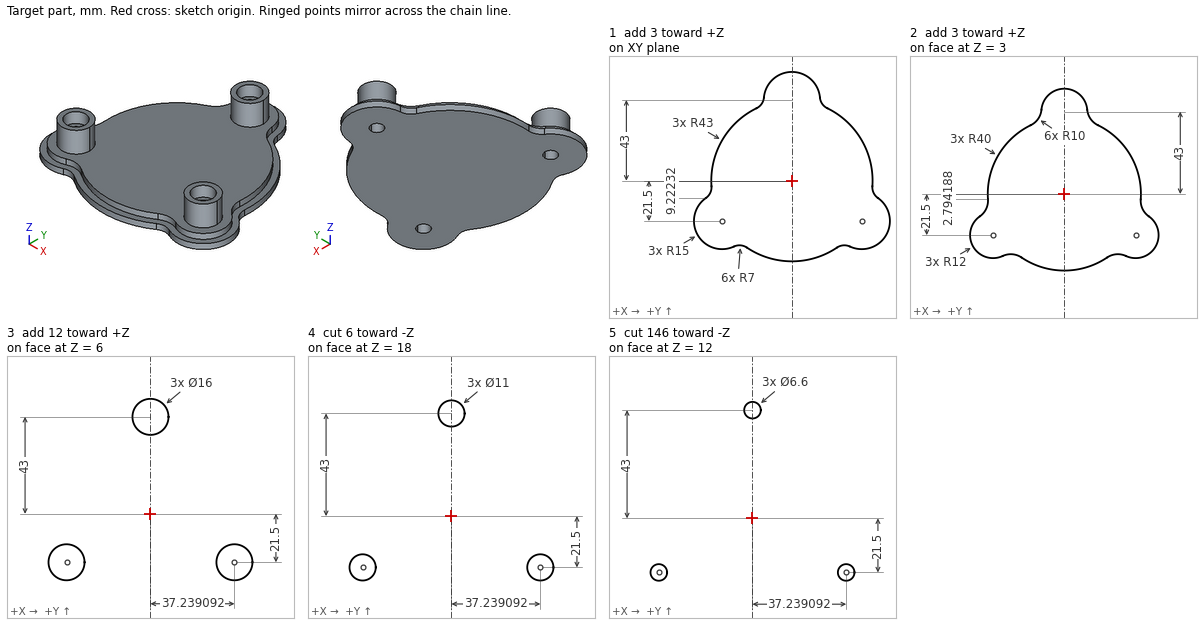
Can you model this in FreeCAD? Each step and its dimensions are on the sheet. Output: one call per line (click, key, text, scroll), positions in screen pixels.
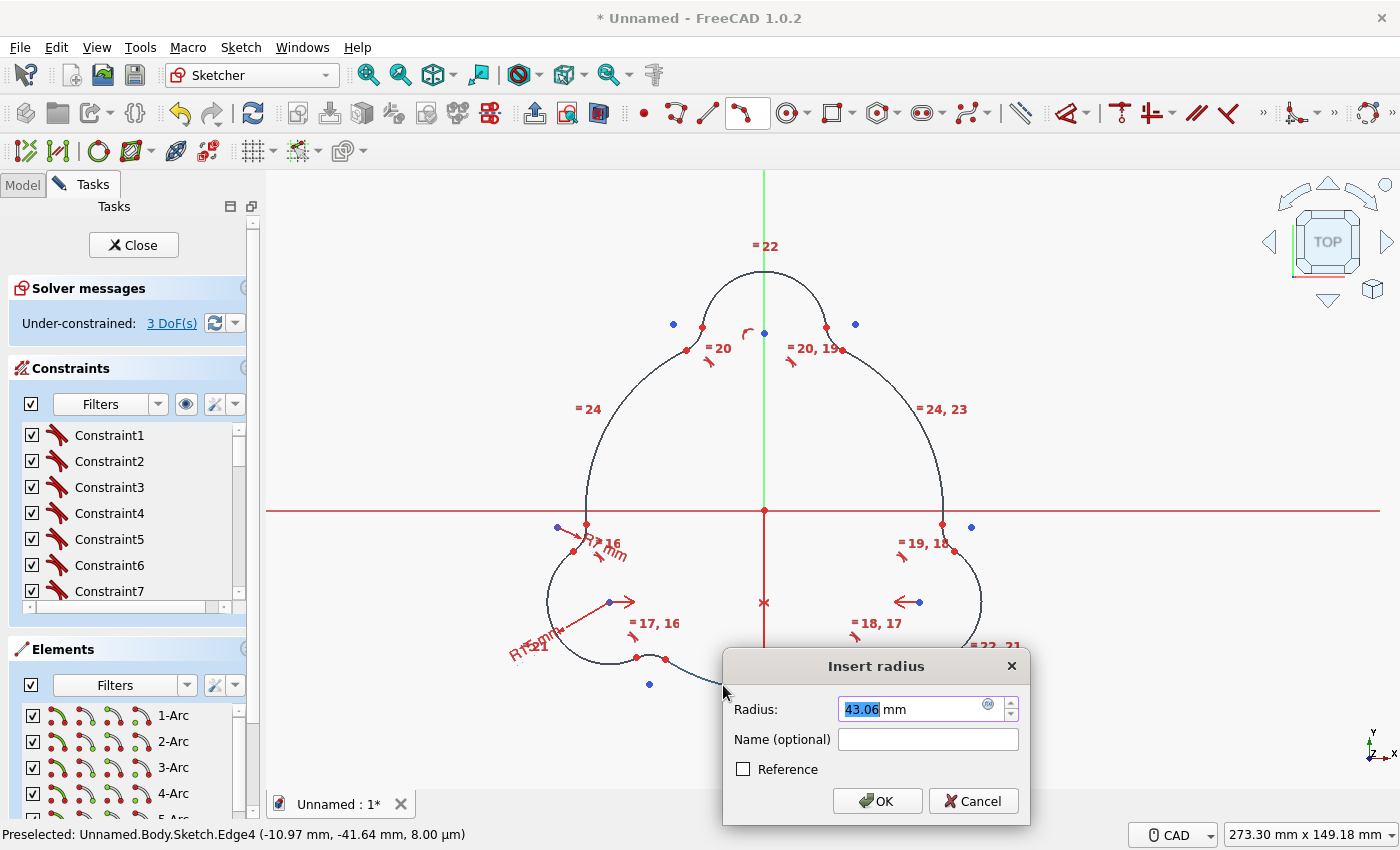
text(43)
key(Return)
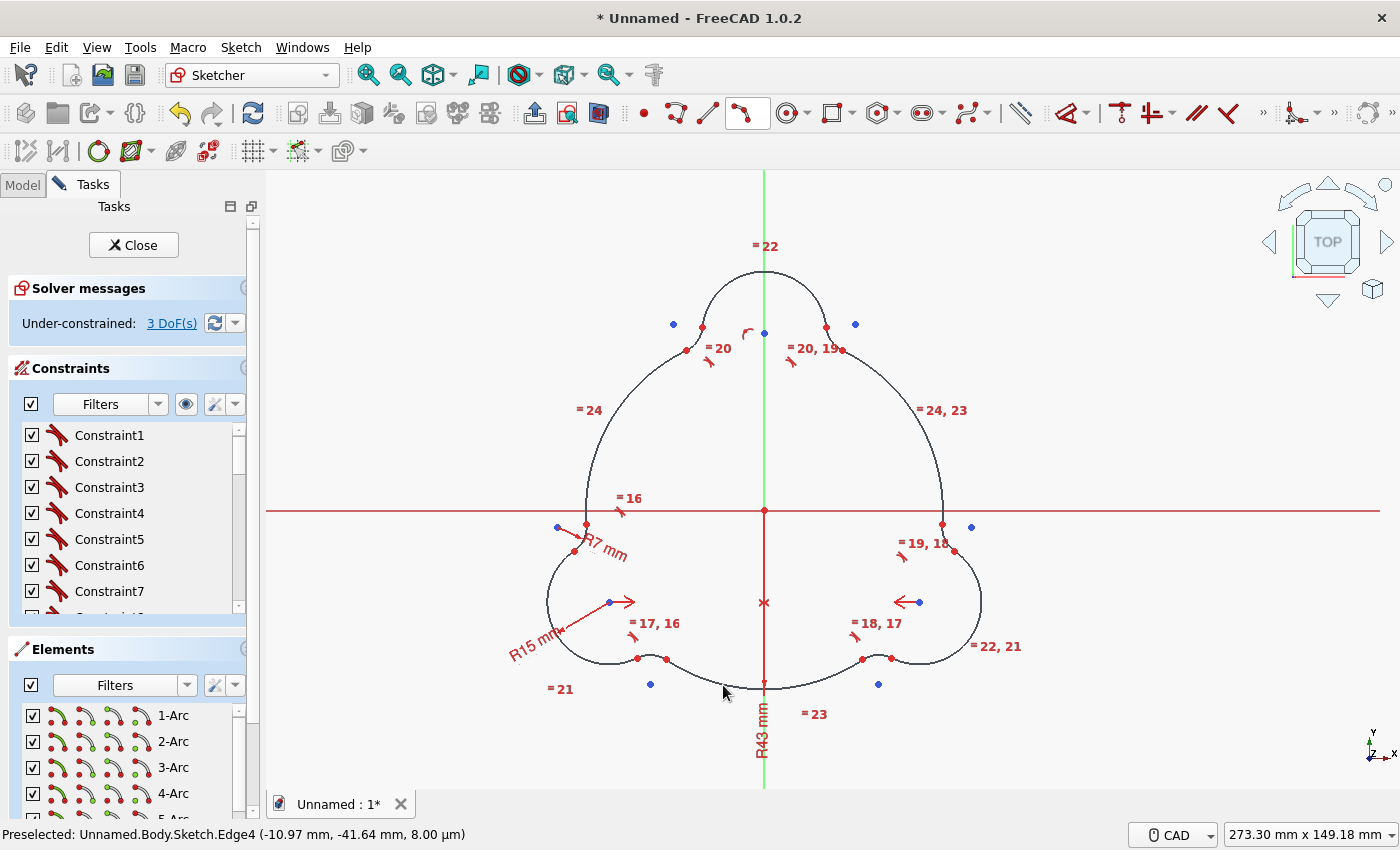
click(764, 334)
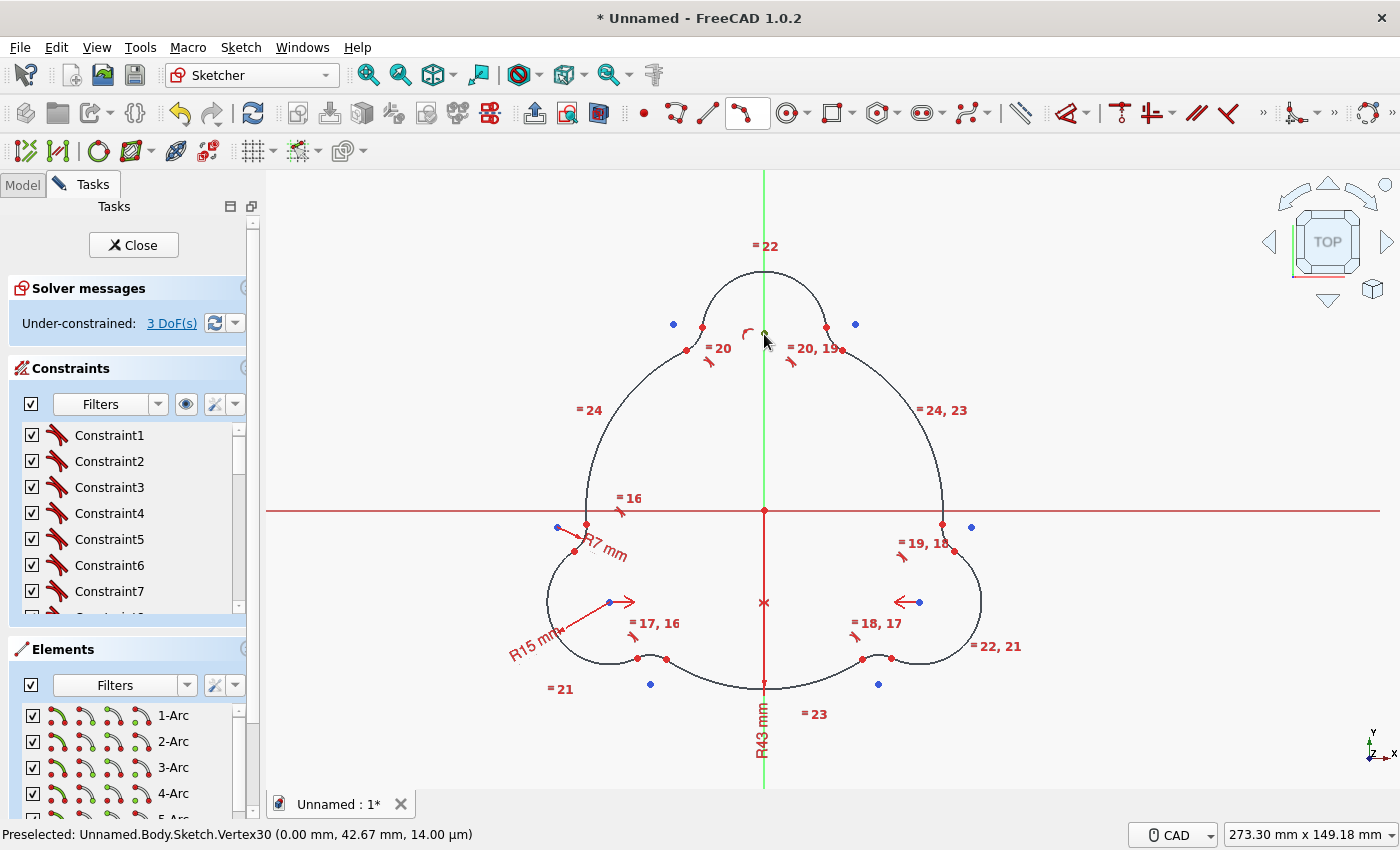
key(i)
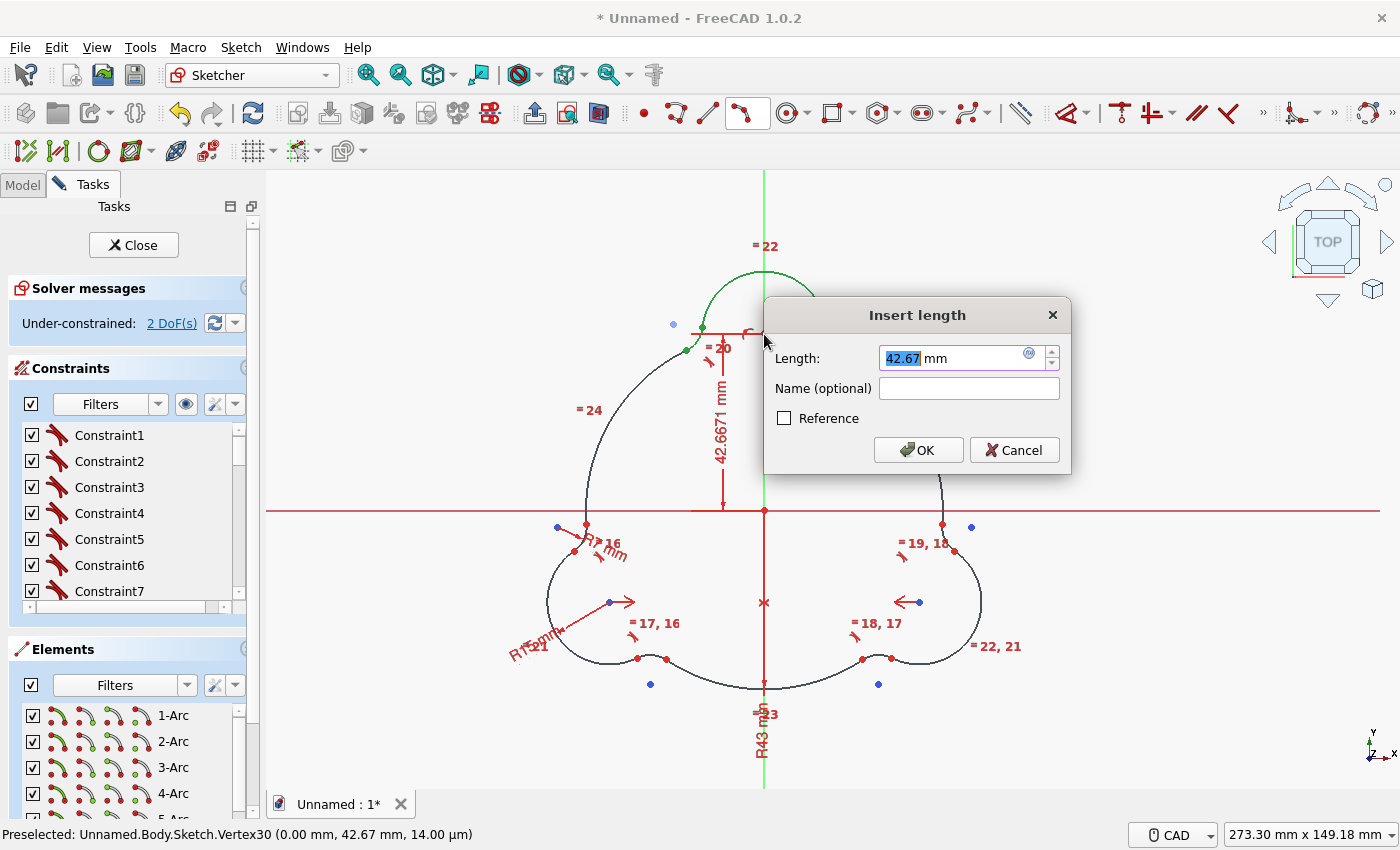
text(43)
key(Return)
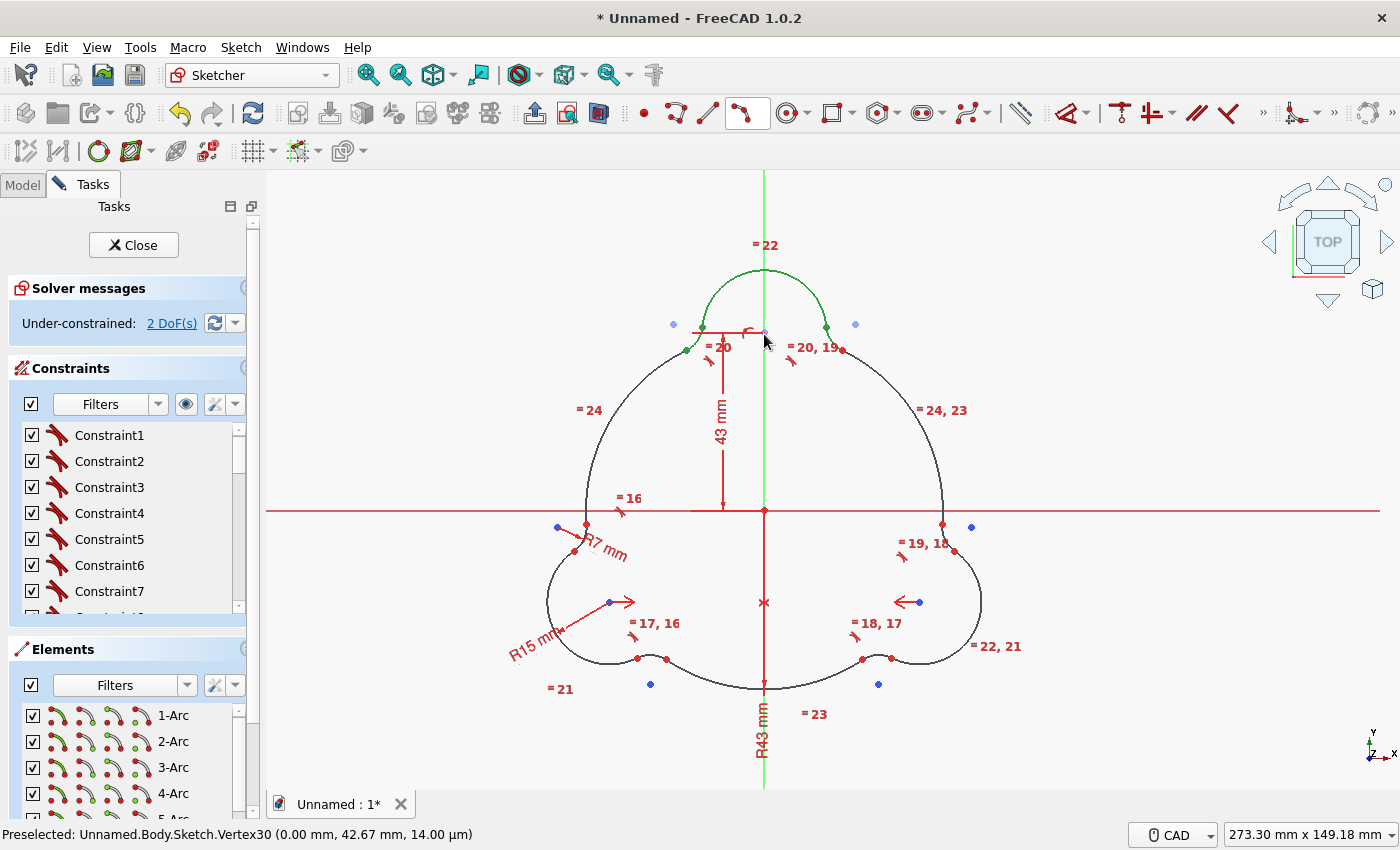
click(610, 602)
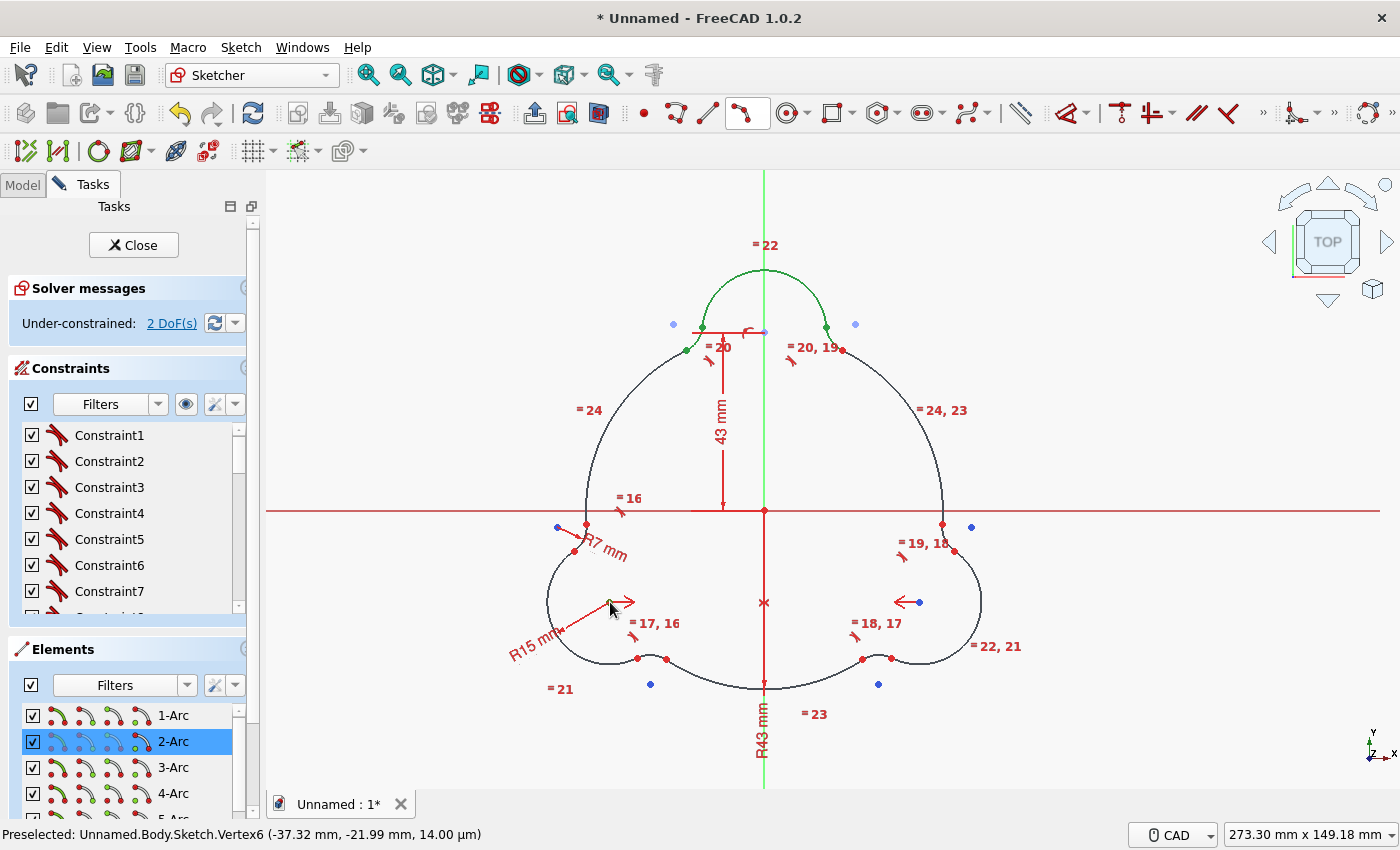
click(1088, 114)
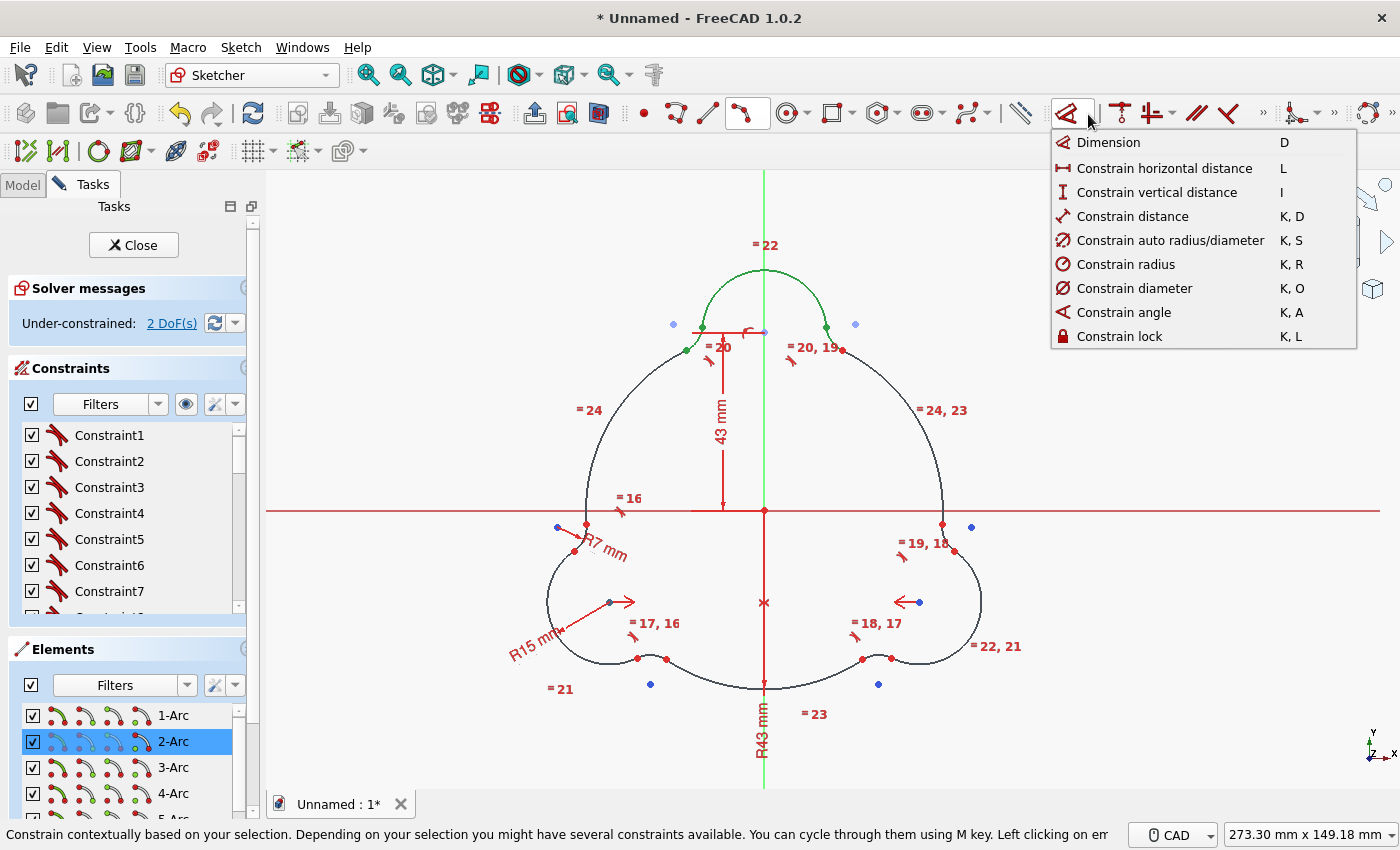
click(1204, 192)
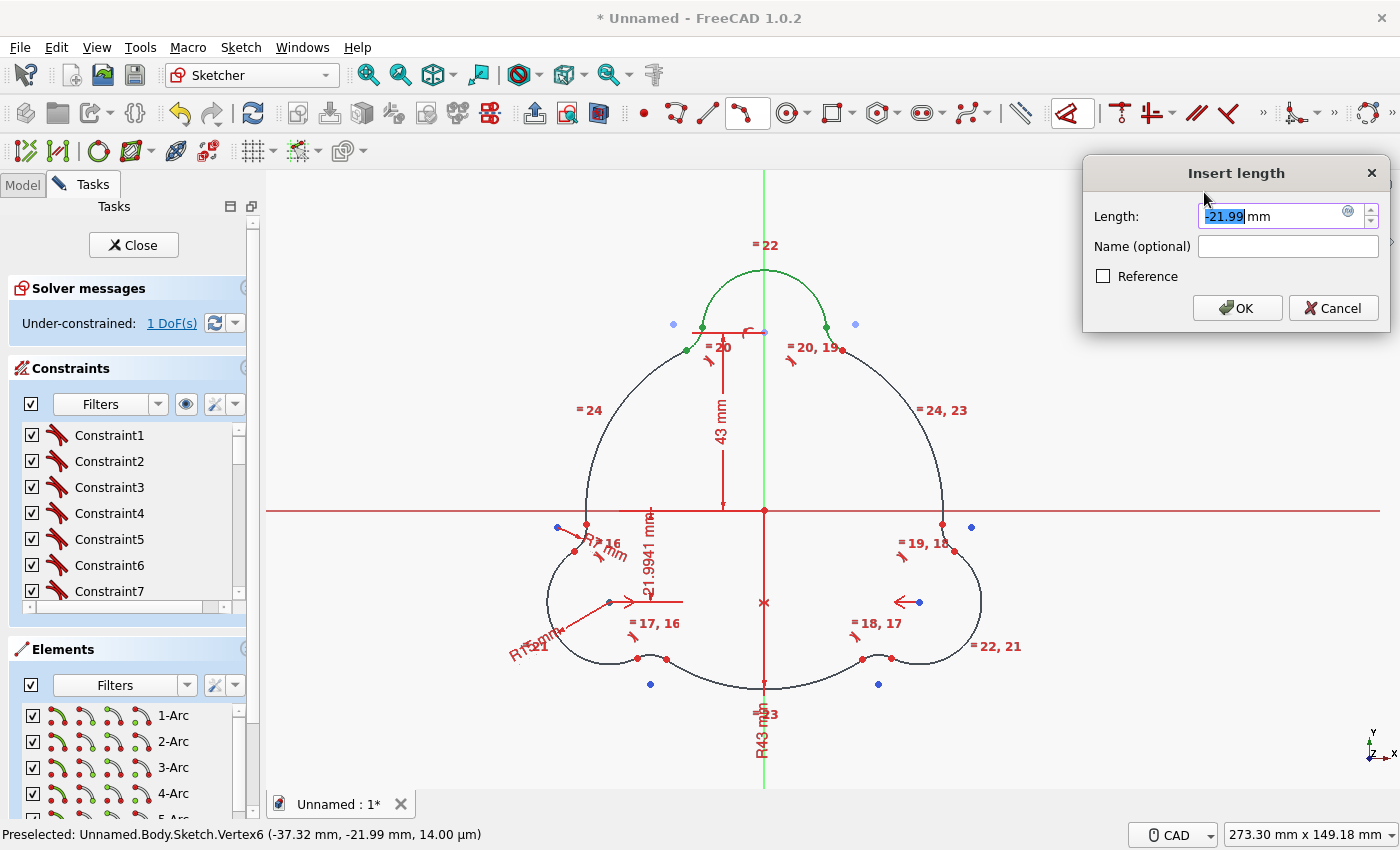
text(-21.5)
key(Return)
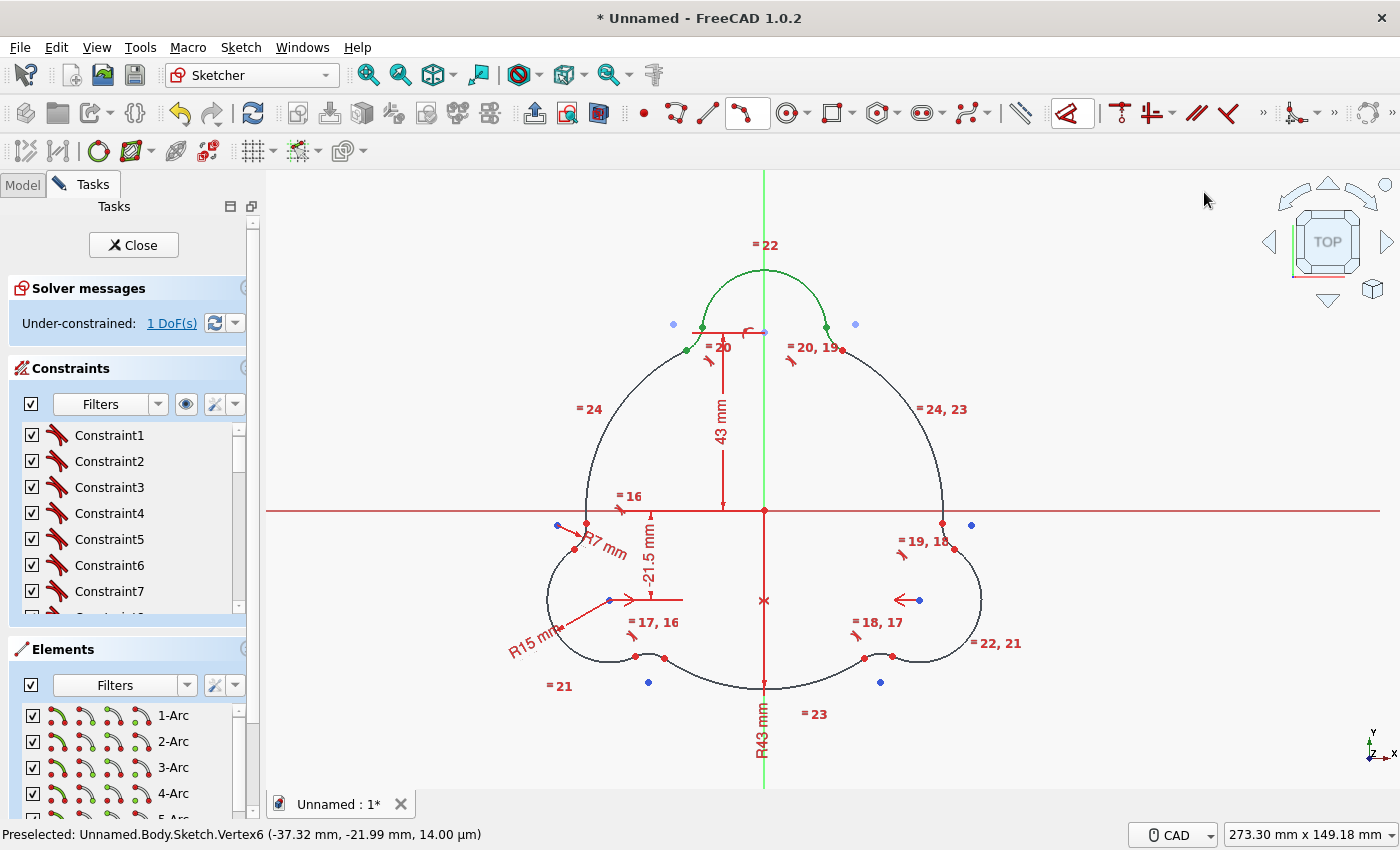
click(574, 549)